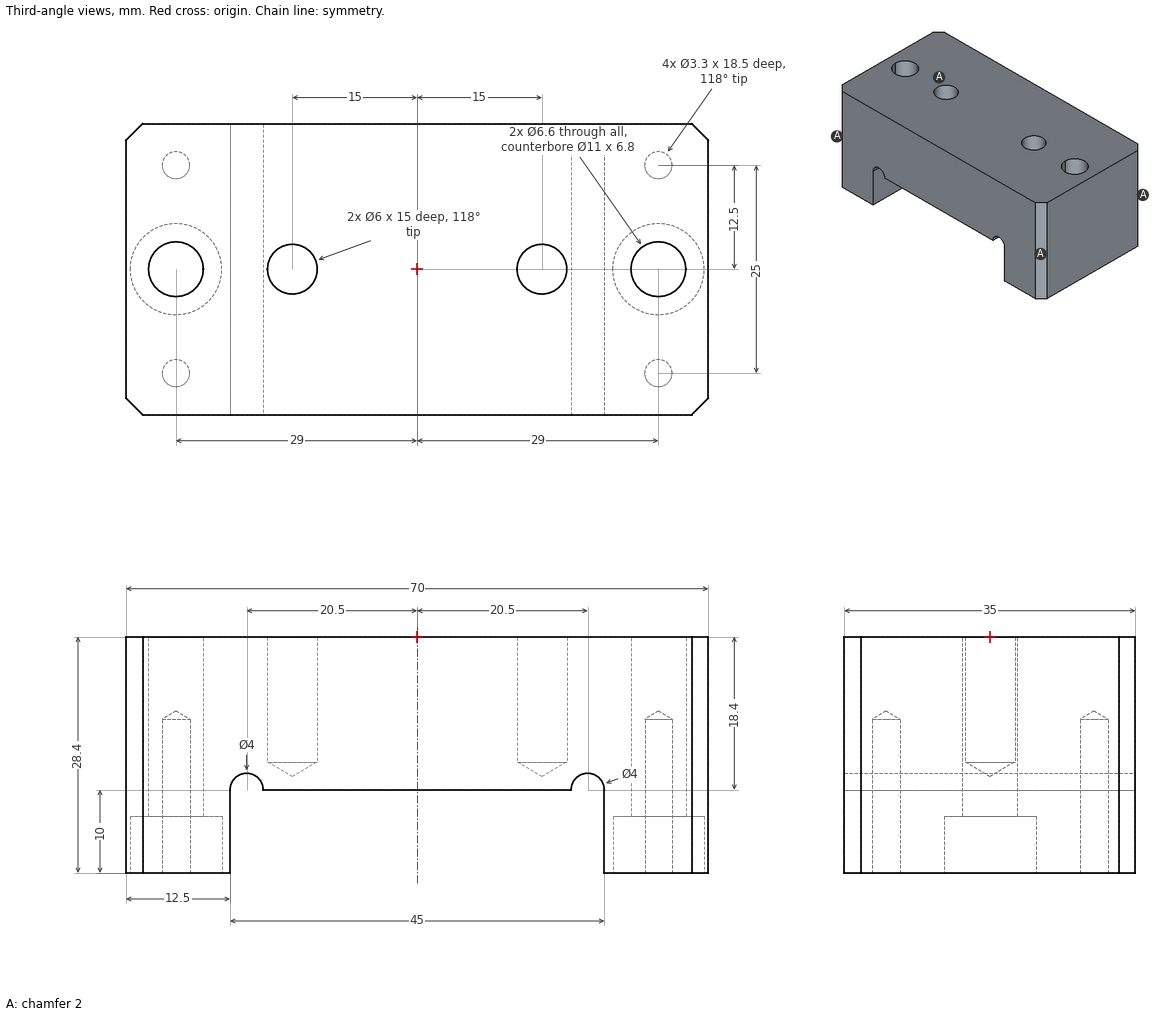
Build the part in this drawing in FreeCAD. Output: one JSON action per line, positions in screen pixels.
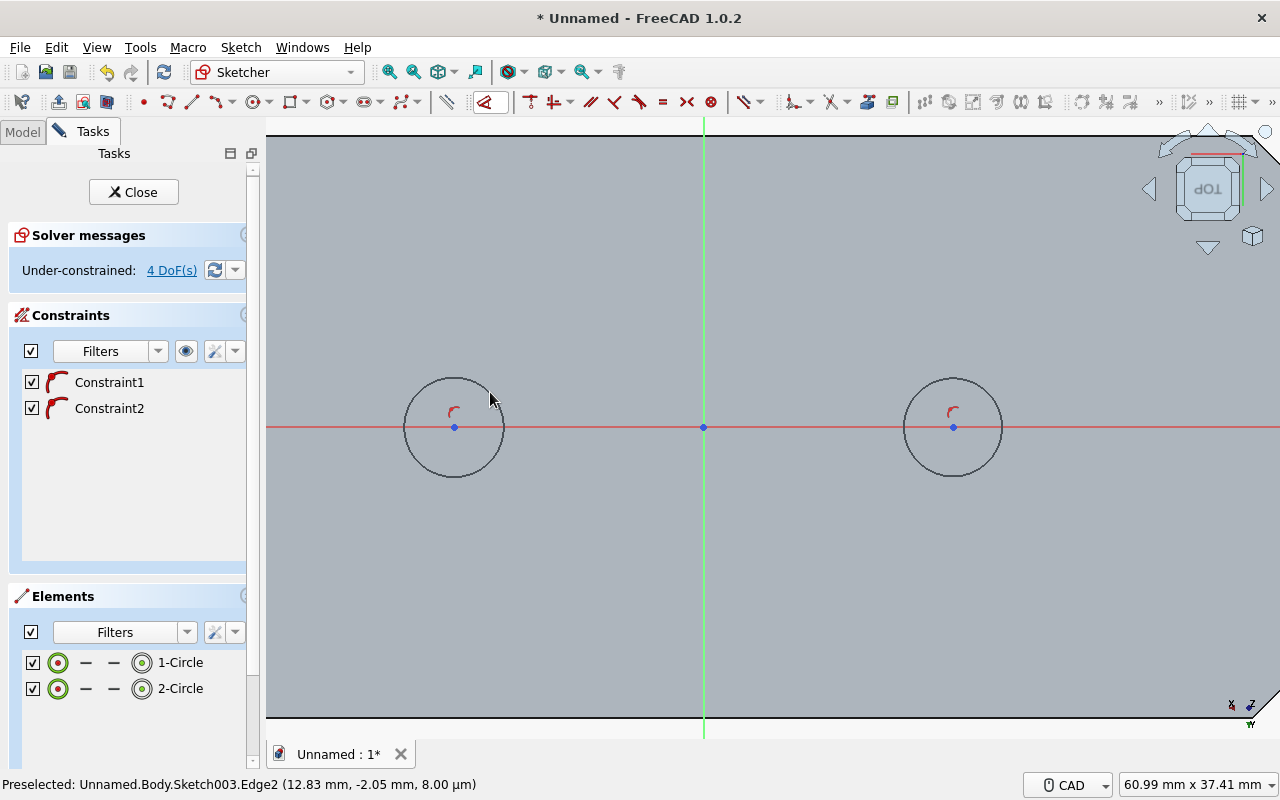
{"action": "left_click", "coordinate": [988, 393]}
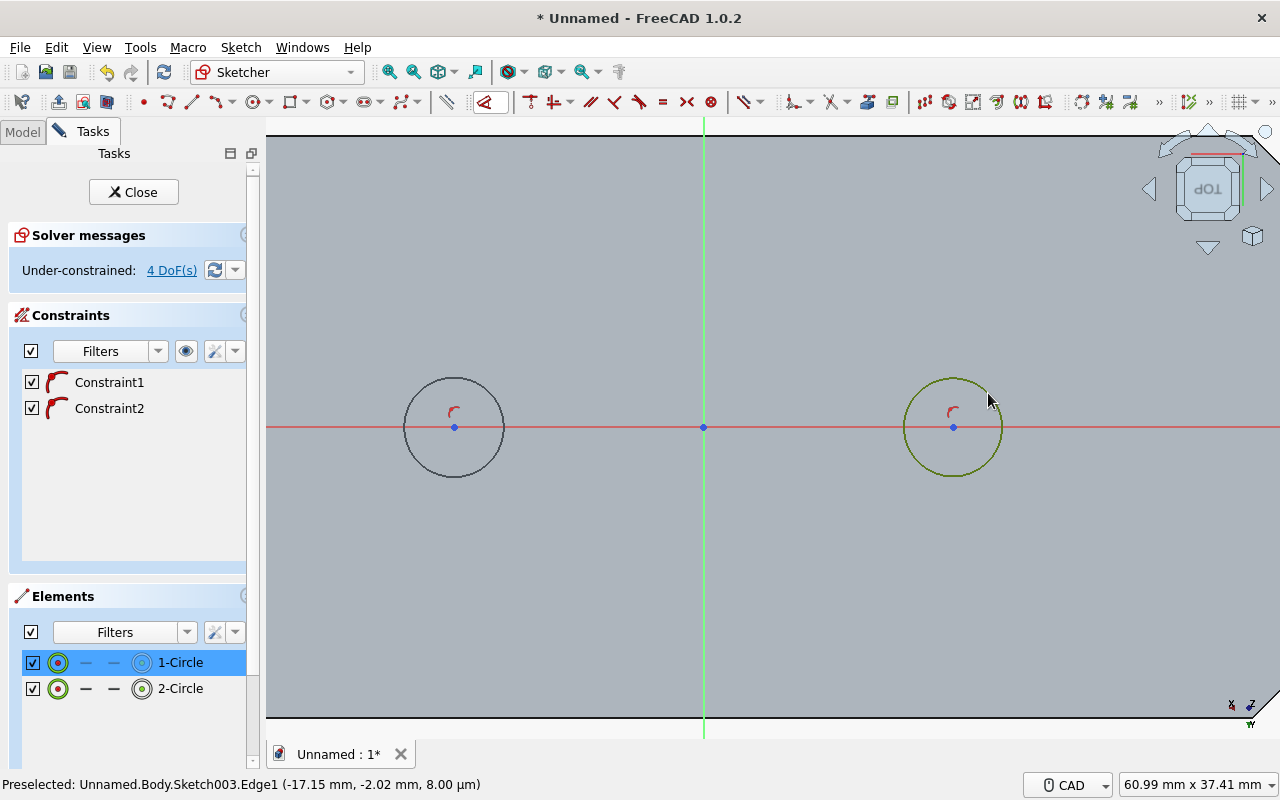
{"action": "left_click", "coordinate": [489, 392]}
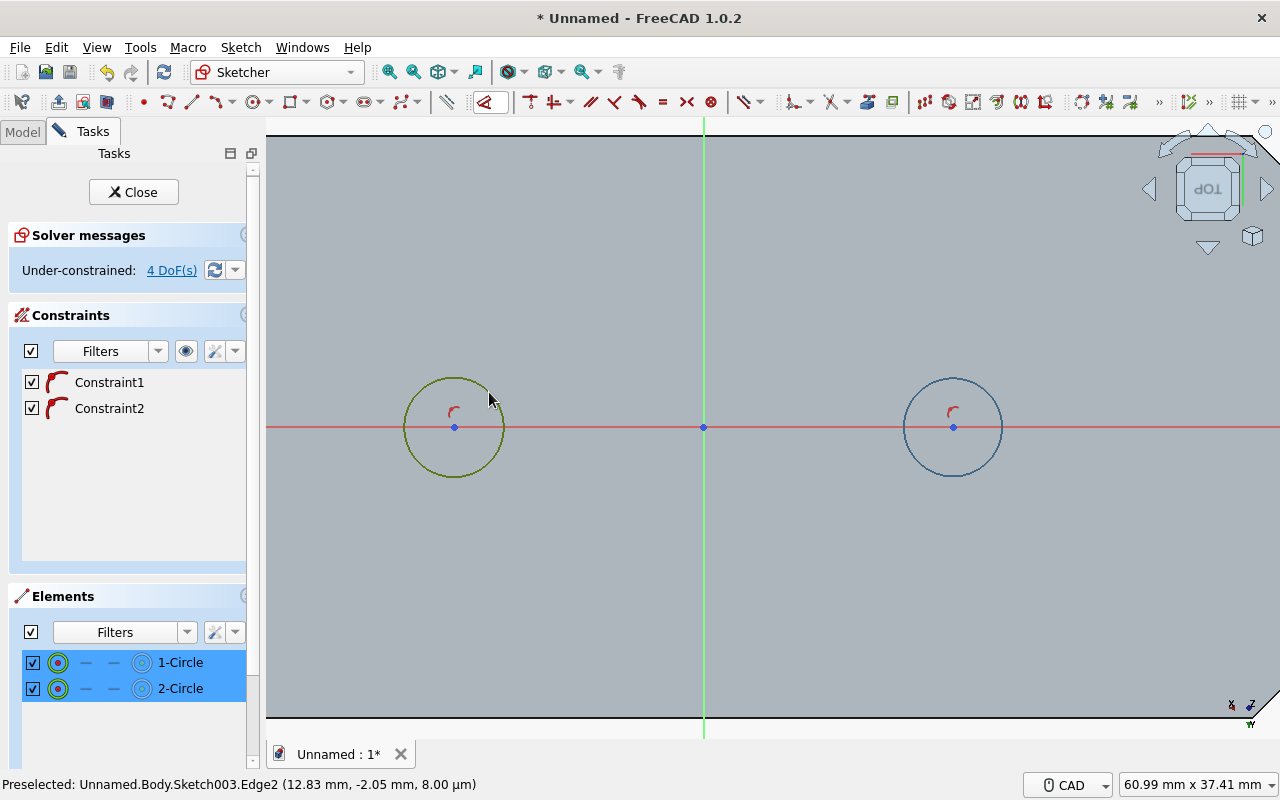
{"action": "key", "text": "e"}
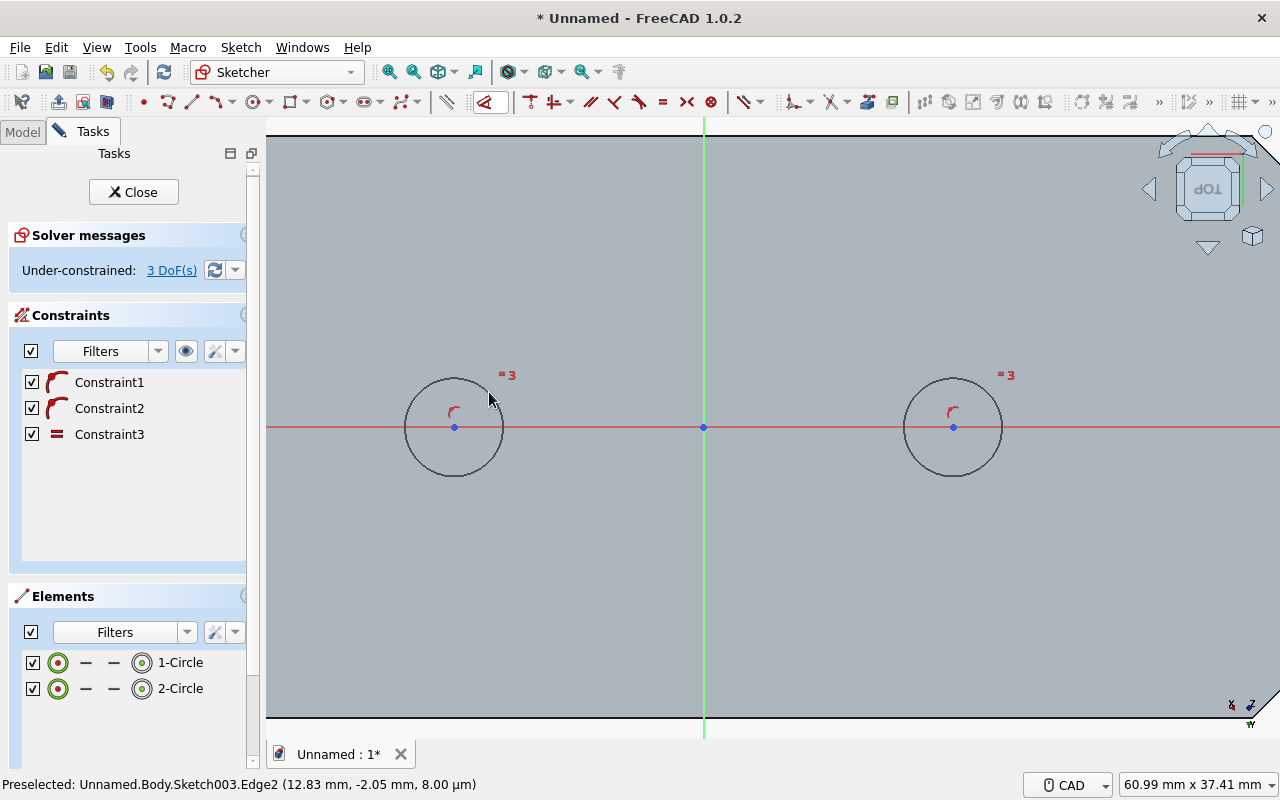
{"action": "key", "text": "d"}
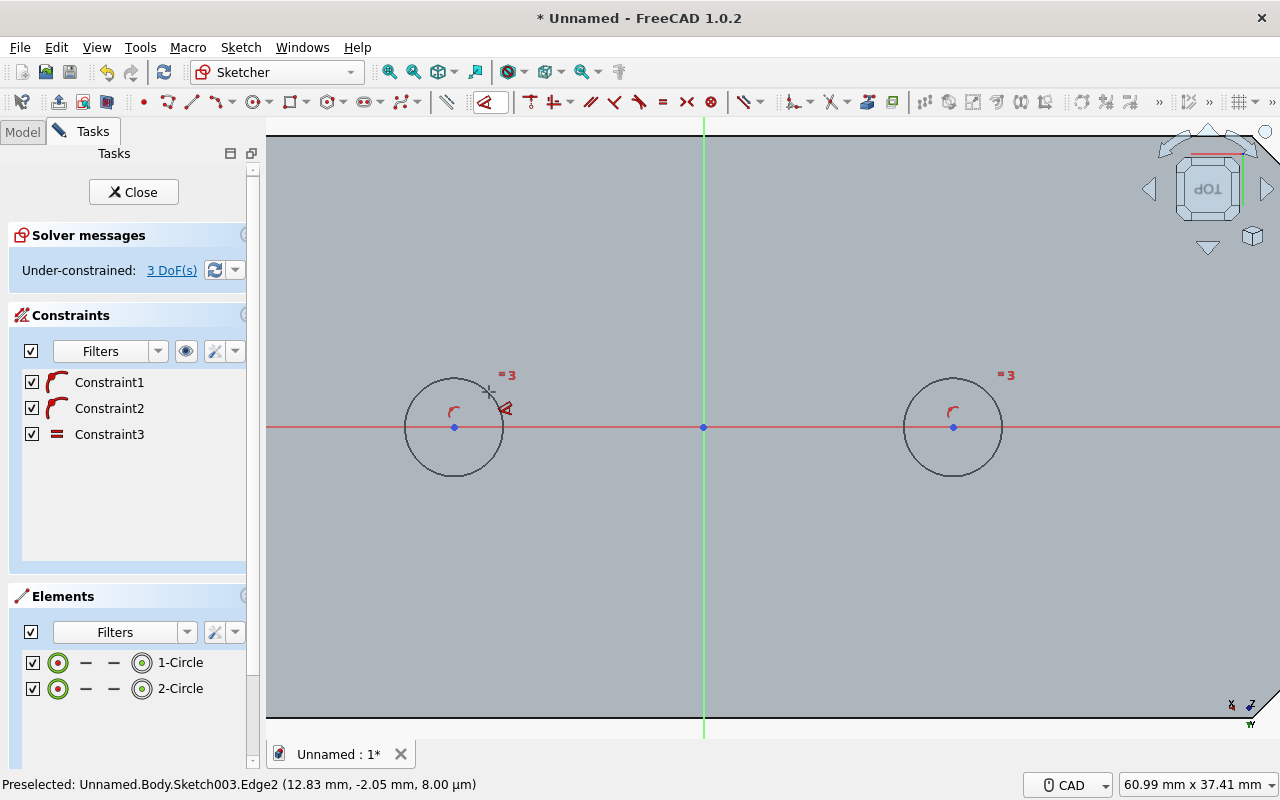
{"action": "left_click", "coordinate": [988, 393]}
{"action": "left_click", "coordinate": [1011, 371]}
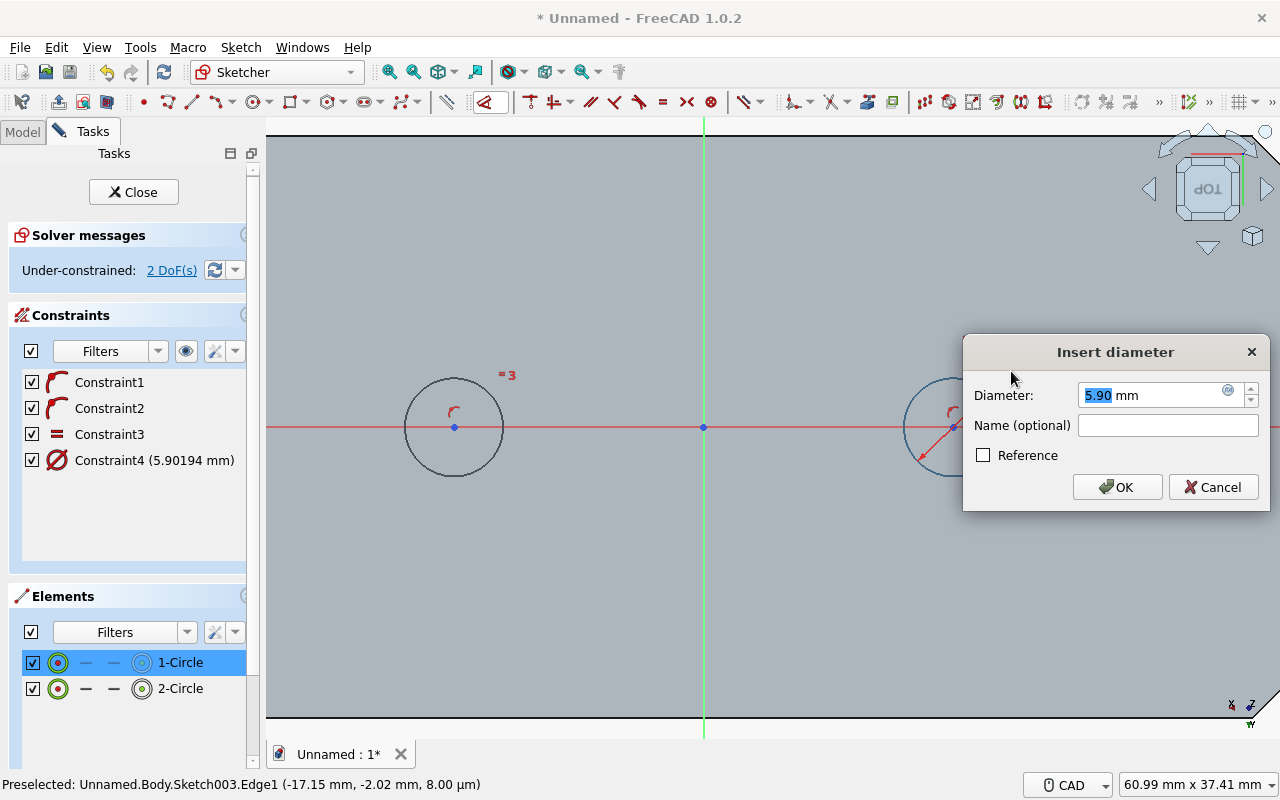
{"action": "type", "text": "6"}
{"action": "key", "text": "Return"}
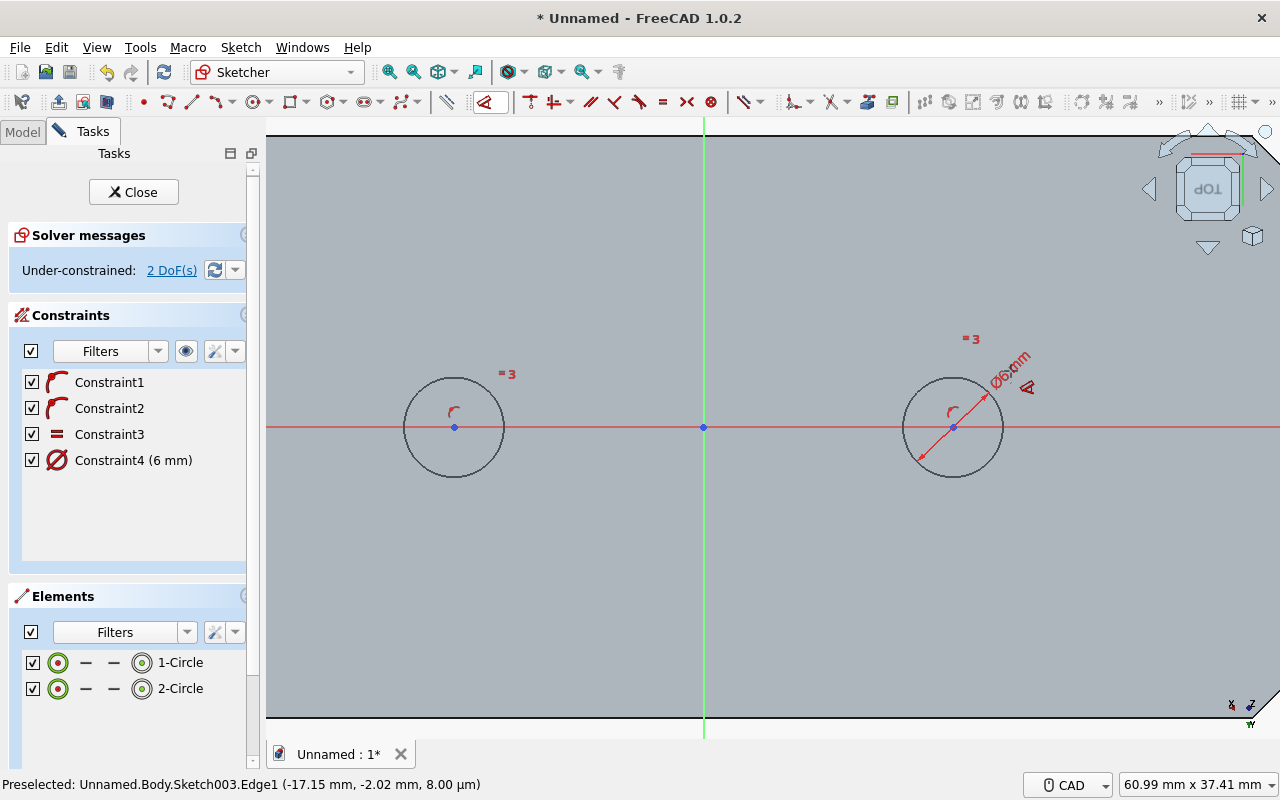
{"action": "left_click", "coordinate": [953, 427]}
{"action": "left_click", "coordinate": [828, 461]}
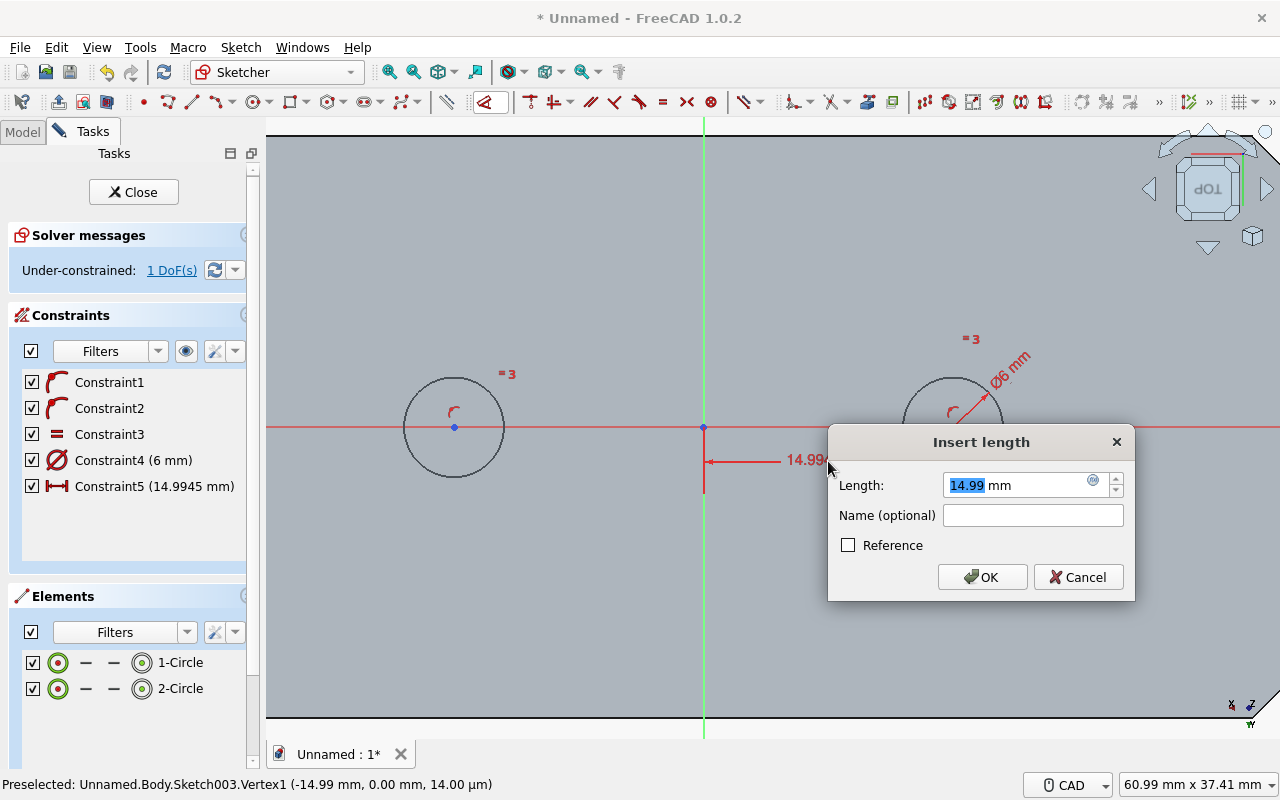
{"action": "type", "text": "15"}
{"action": "key", "text": "Return"}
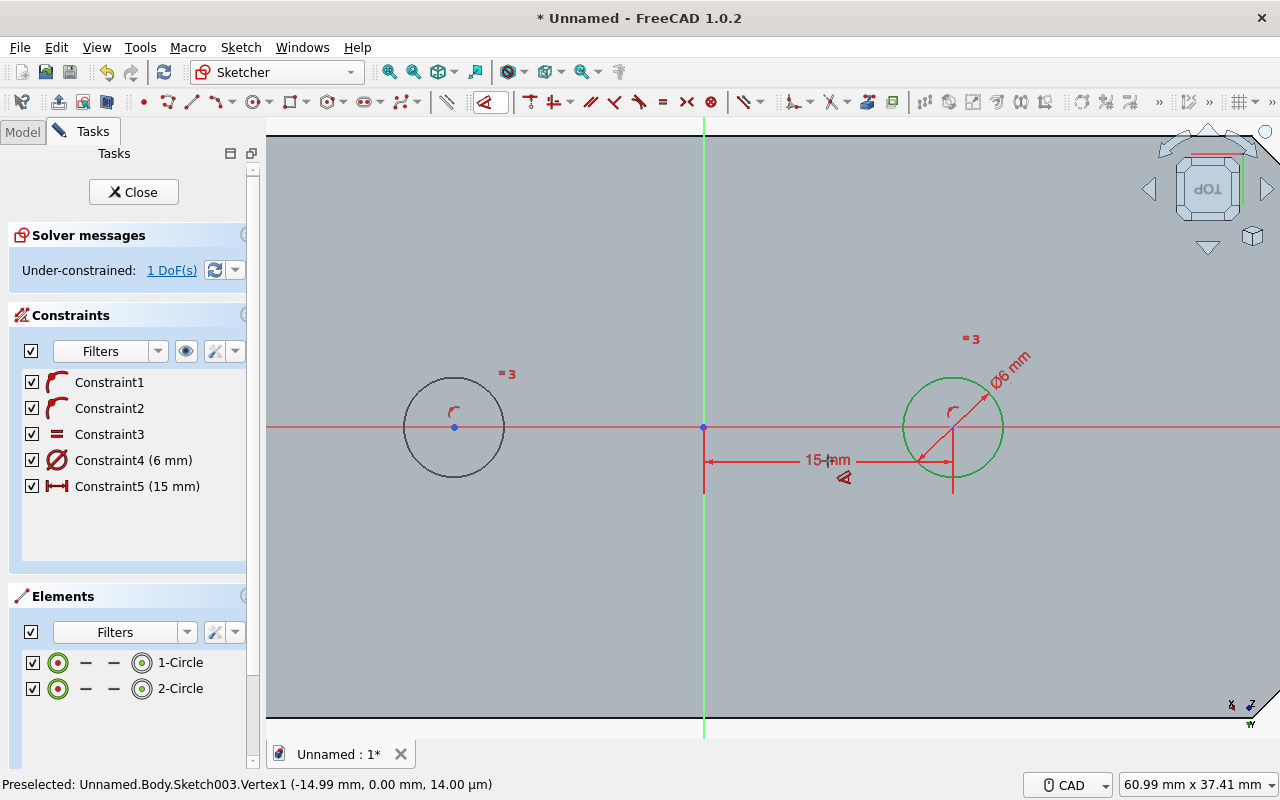
{"action": "left_click", "coordinate": [454, 427]}
{"action": "left_click", "coordinate": [579, 461]}